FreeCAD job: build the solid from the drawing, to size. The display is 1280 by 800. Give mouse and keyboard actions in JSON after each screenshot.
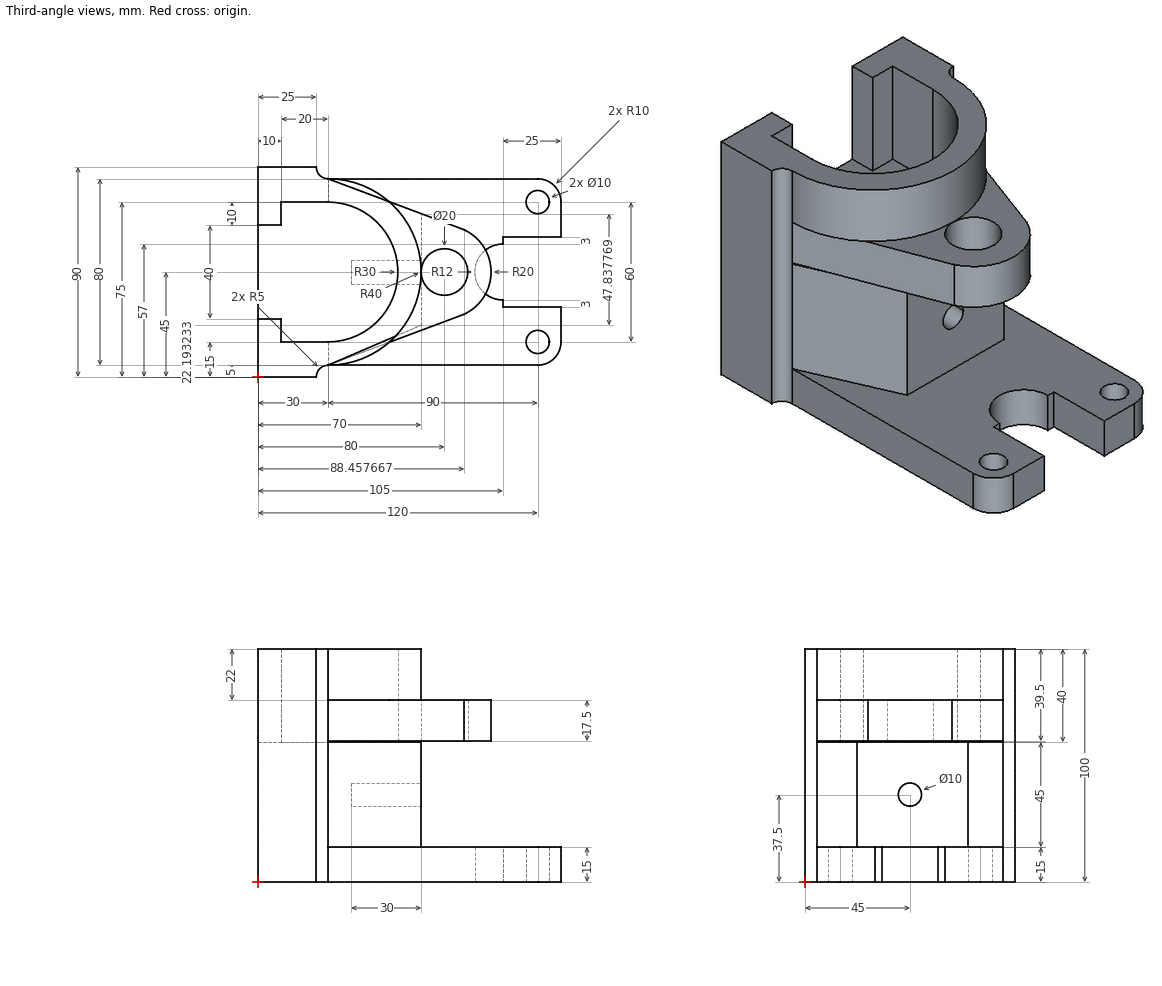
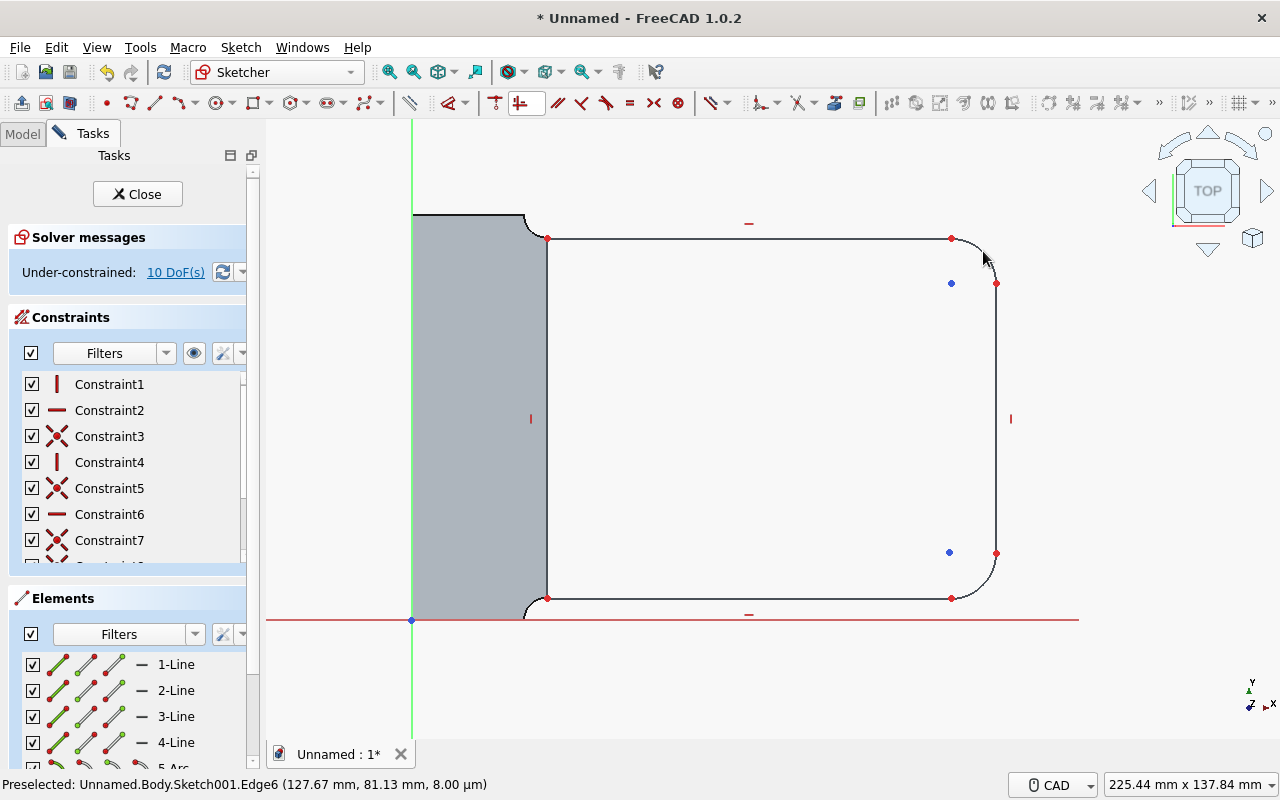
{"action": "left_click", "coordinate": [996, 365]}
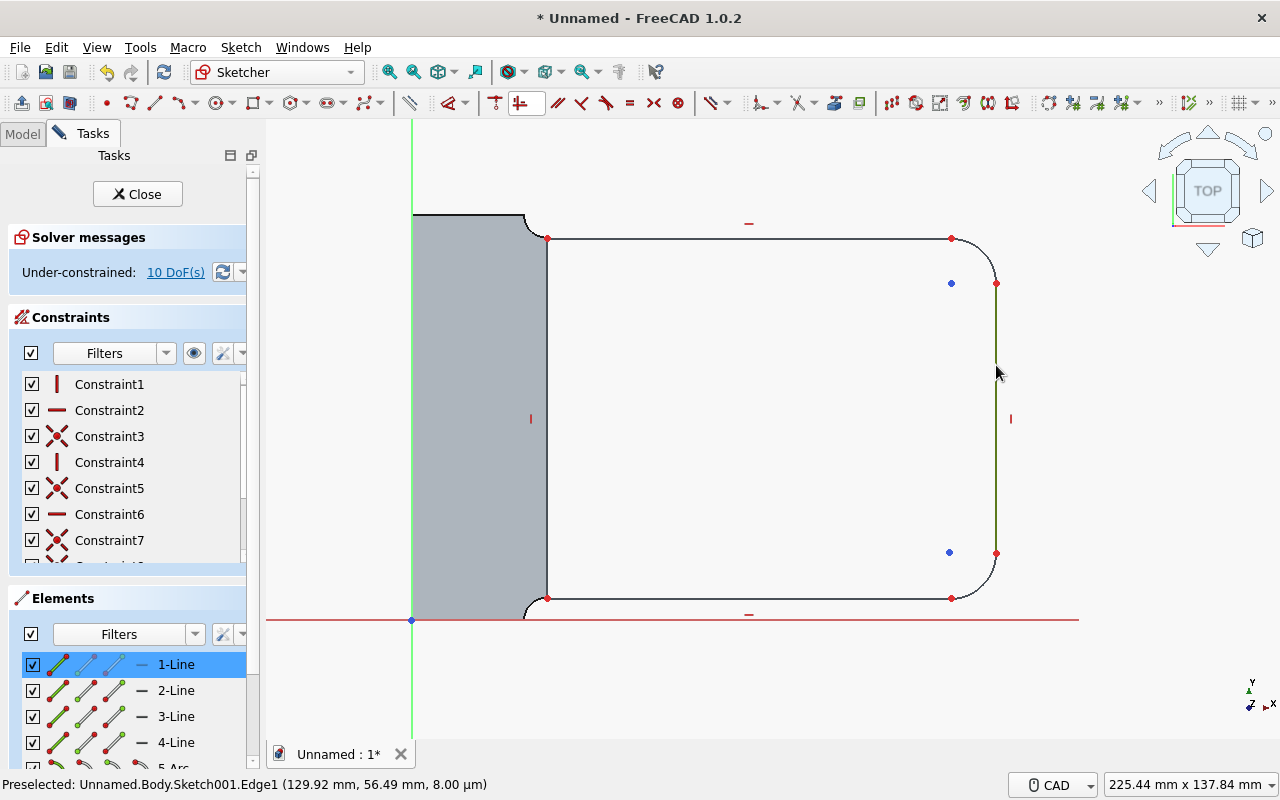
{"action": "left_click", "coordinate": [971, 594]}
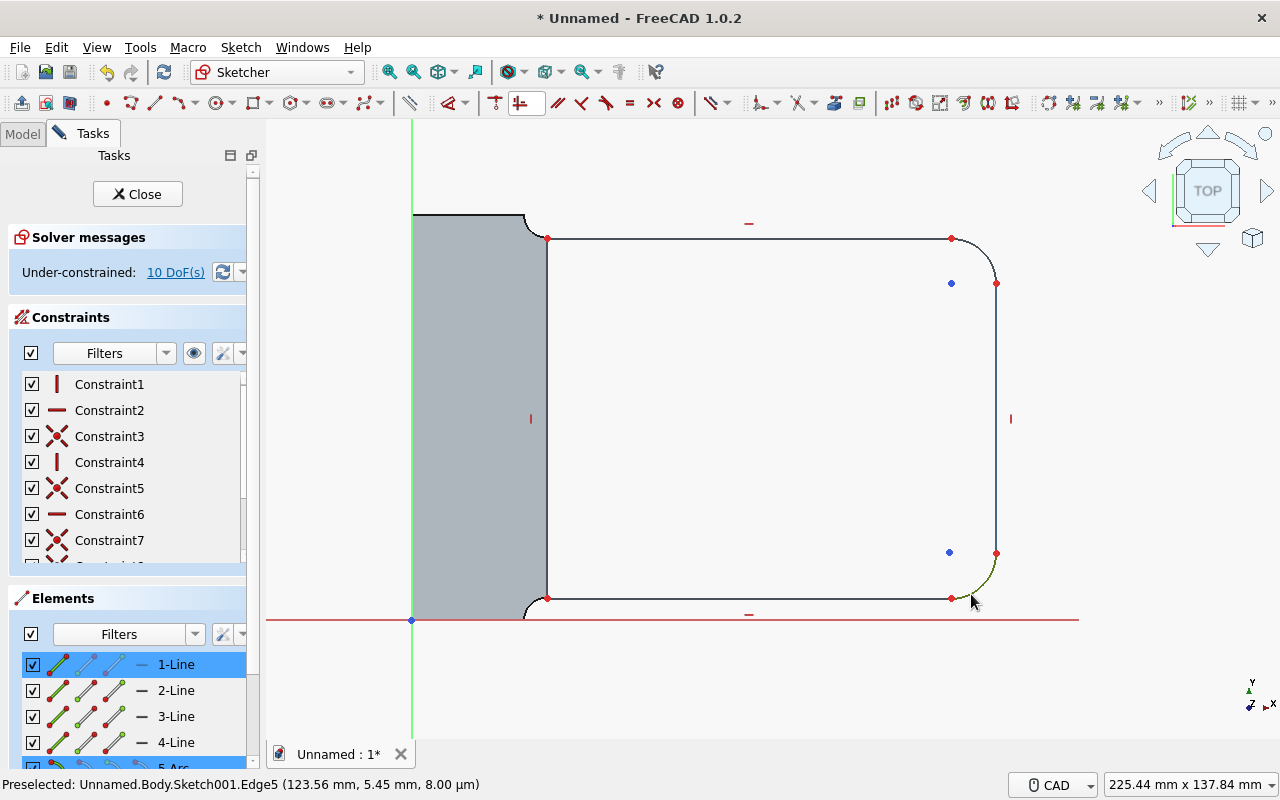
{"action": "left_click", "coordinate": [606, 104]}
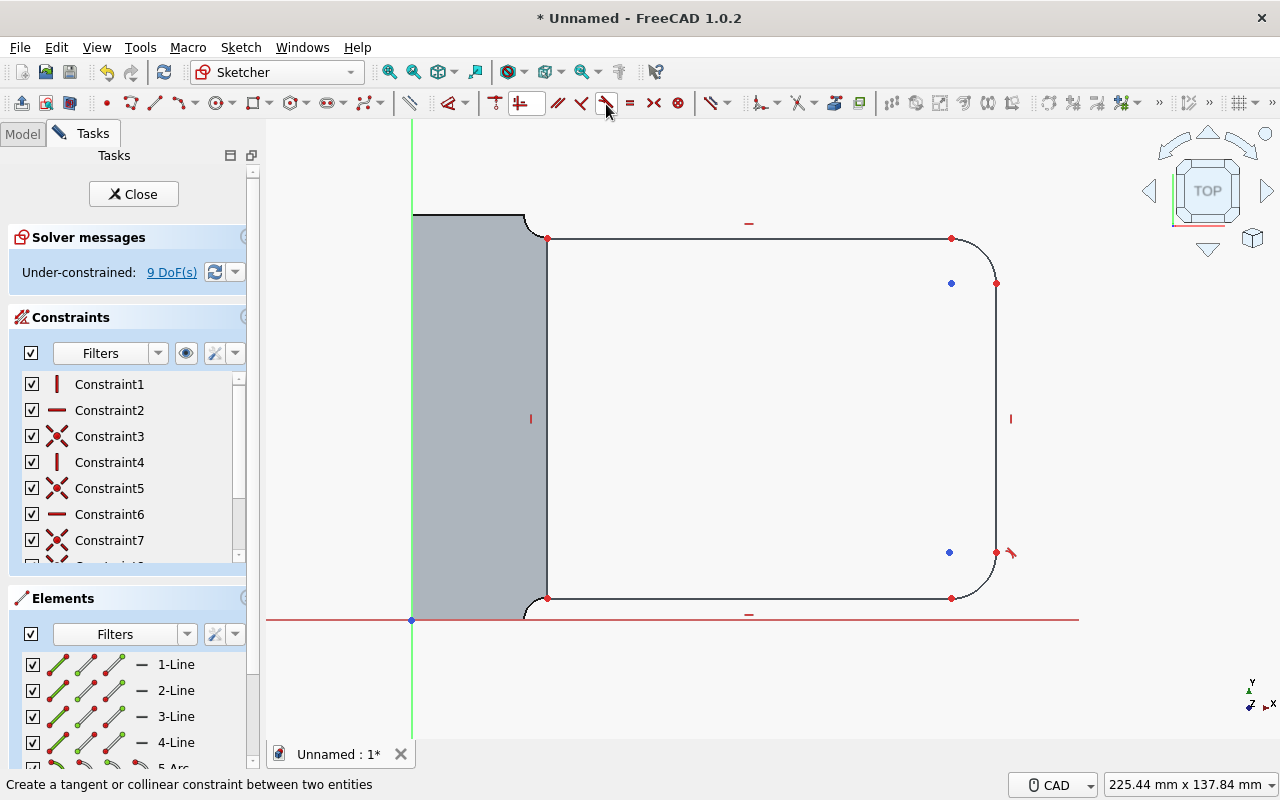
{"action": "left_click", "coordinate": [996, 365]}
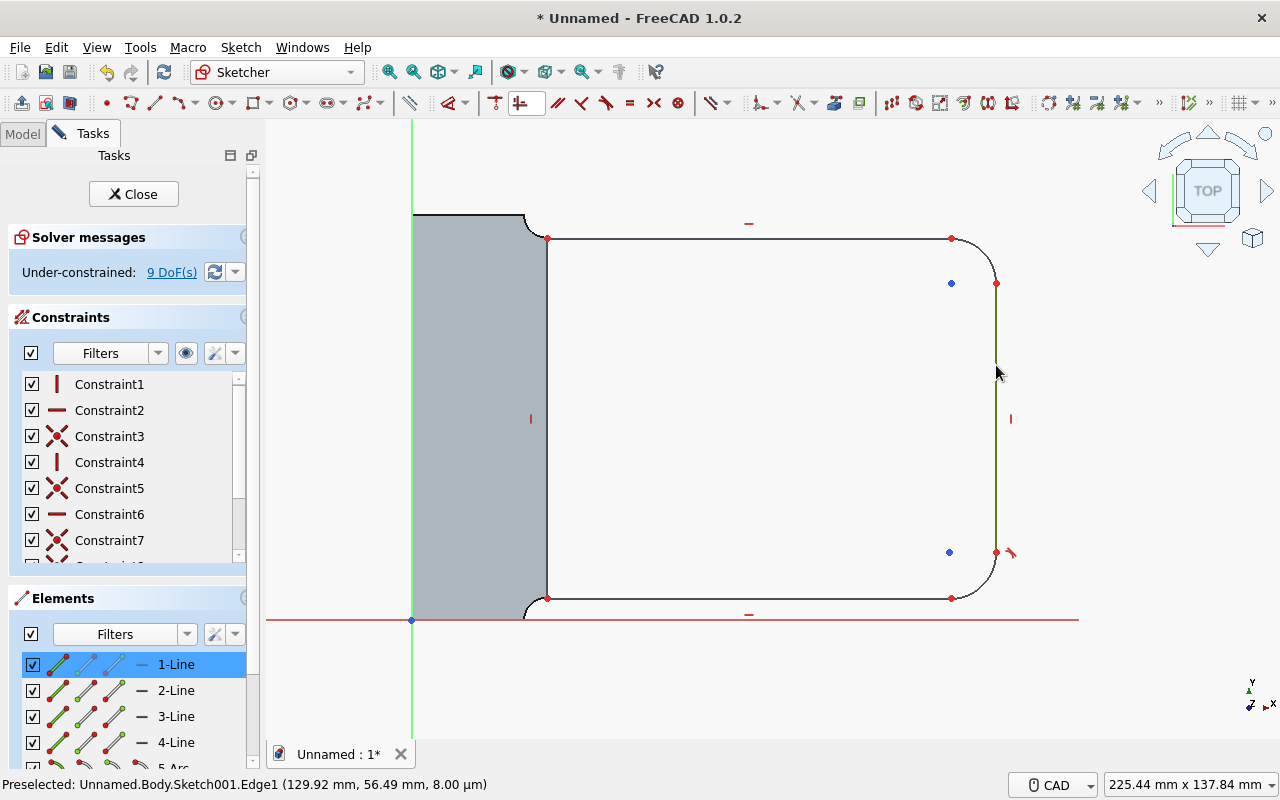
{"action": "left_click", "coordinate": [991, 263]}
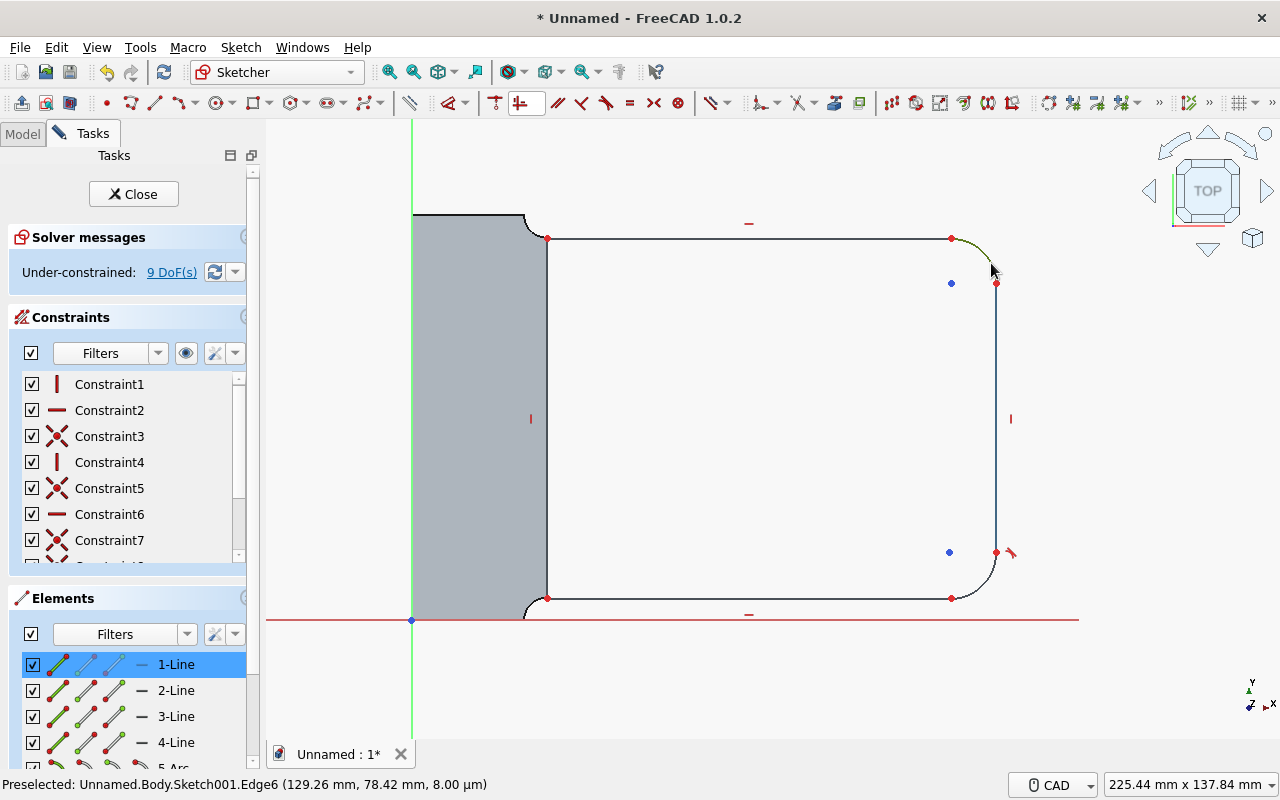
{"action": "left_click", "coordinate": [606, 104]}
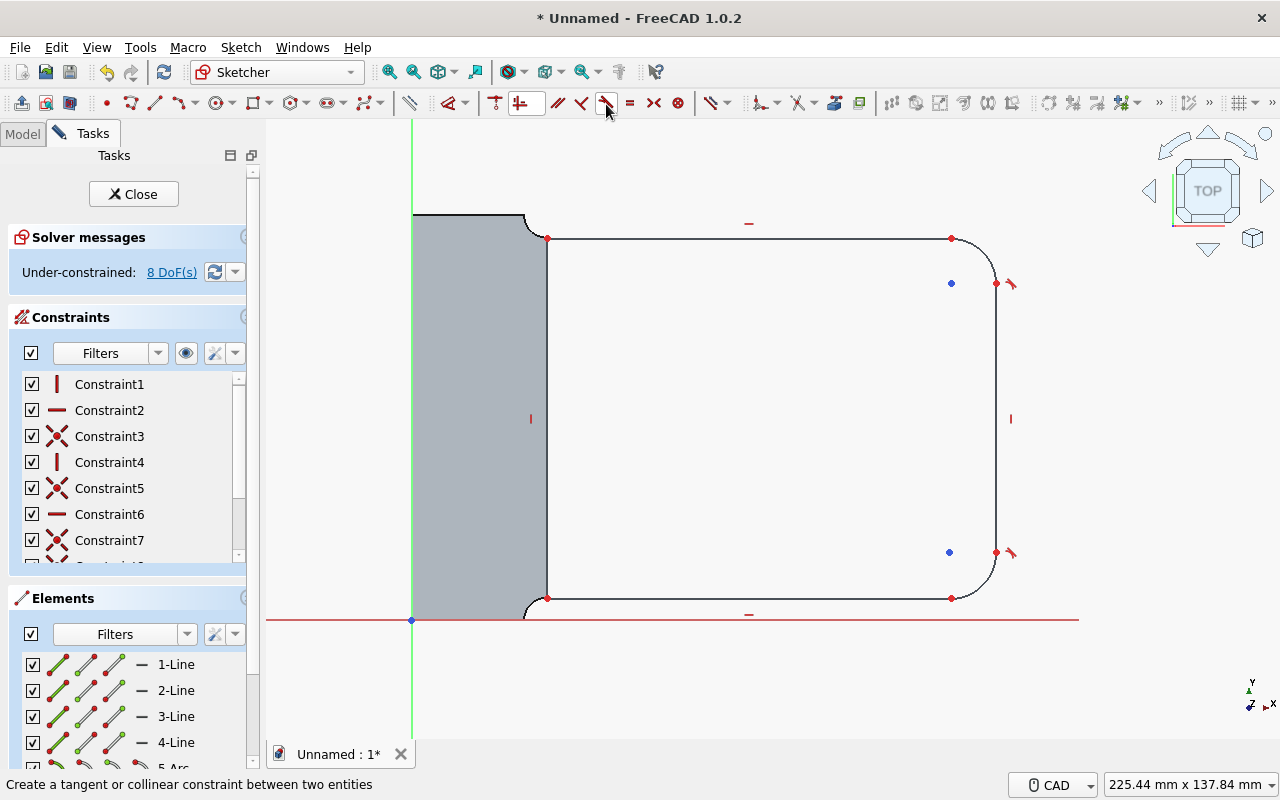
{"action": "left_click", "coordinate": [830, 599]}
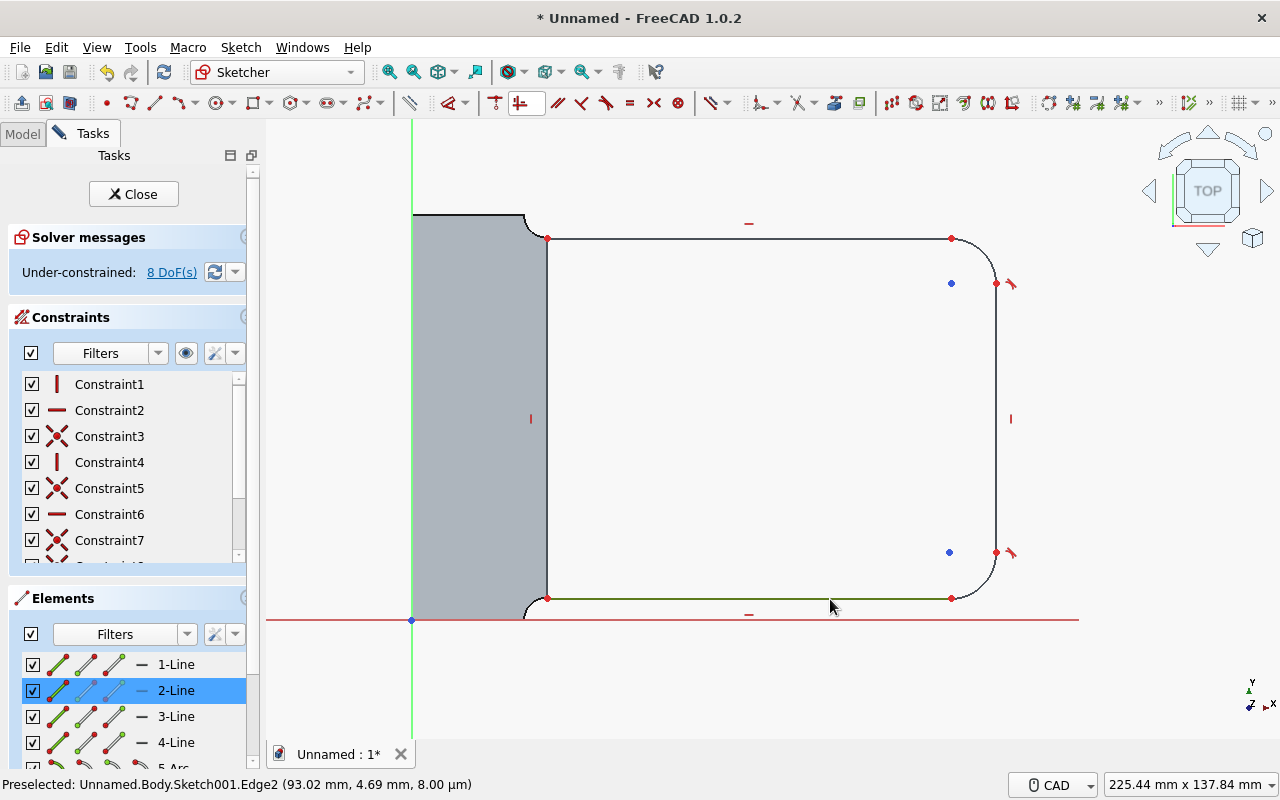
{"action": "left_click", "coordinate": [972, 594]}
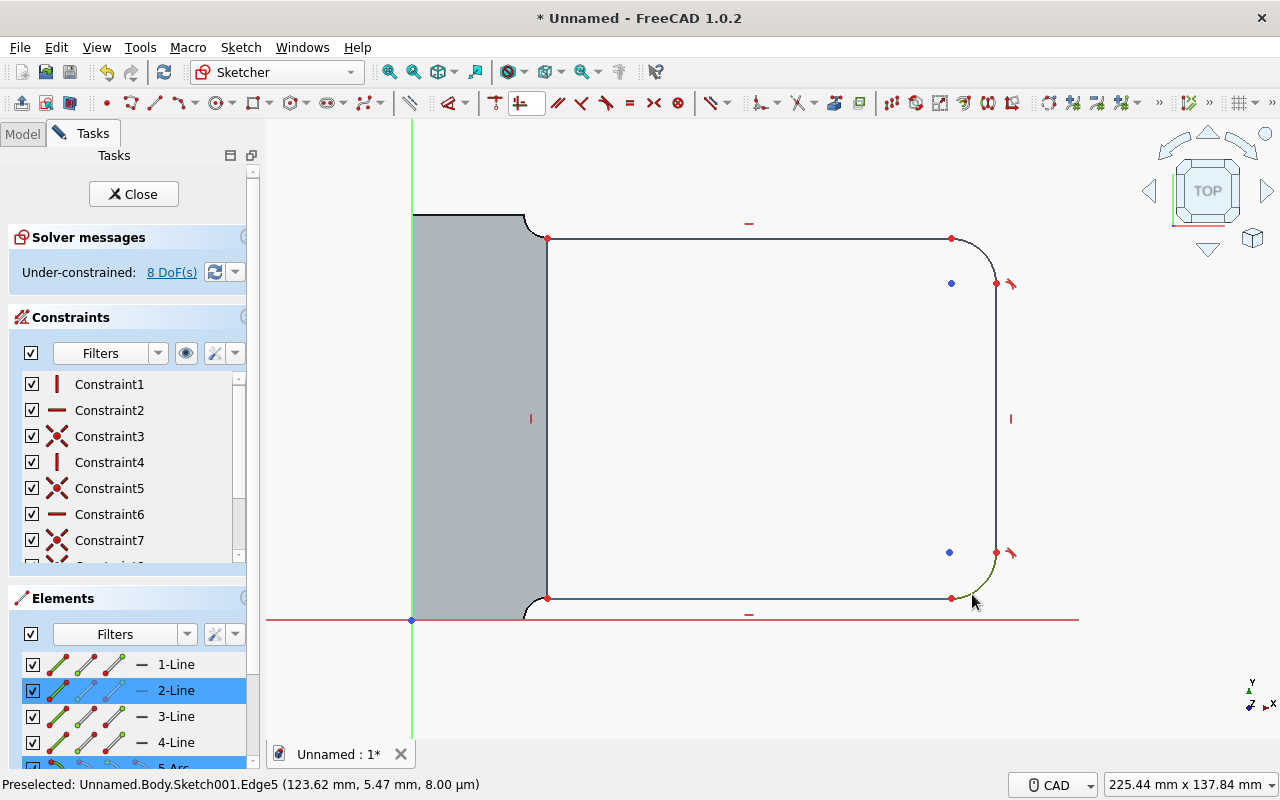
{"action": "key", "text": "t"}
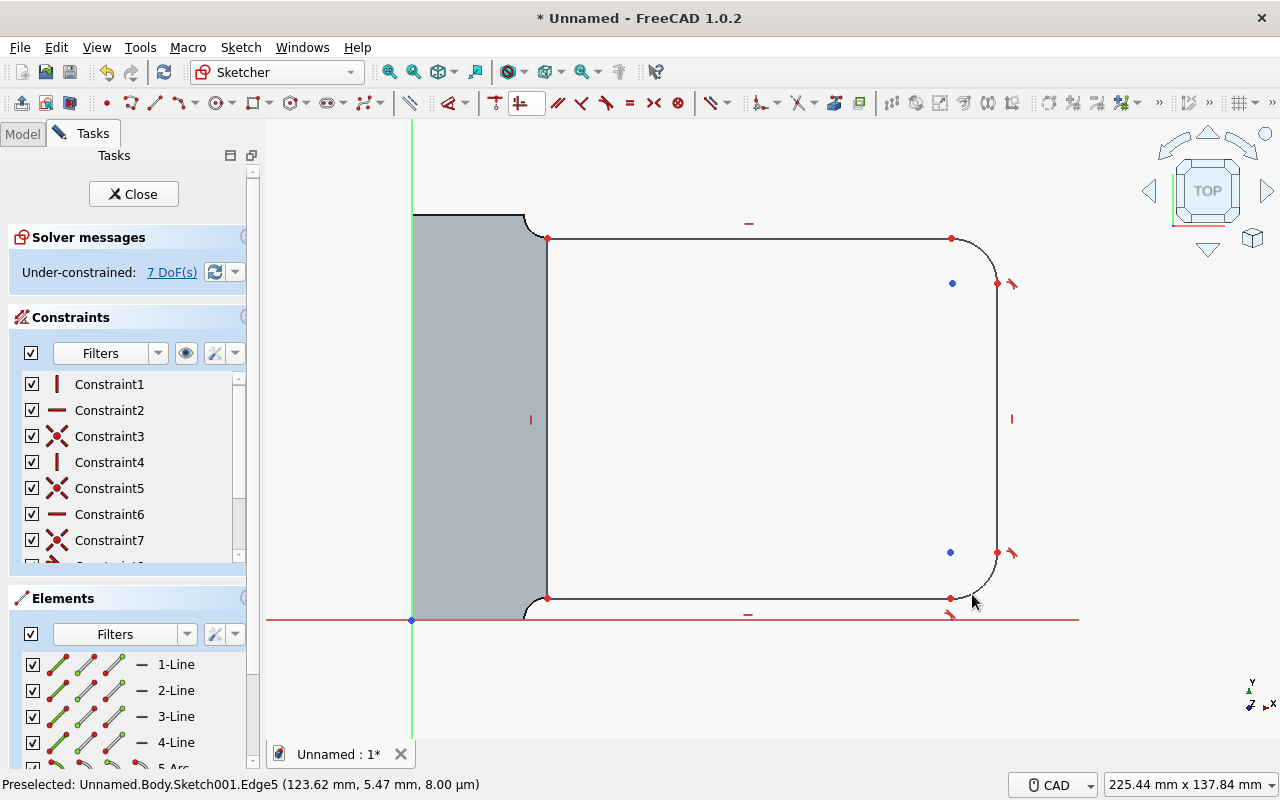
{"action": "left_click", "coordinate": [668, 239]}